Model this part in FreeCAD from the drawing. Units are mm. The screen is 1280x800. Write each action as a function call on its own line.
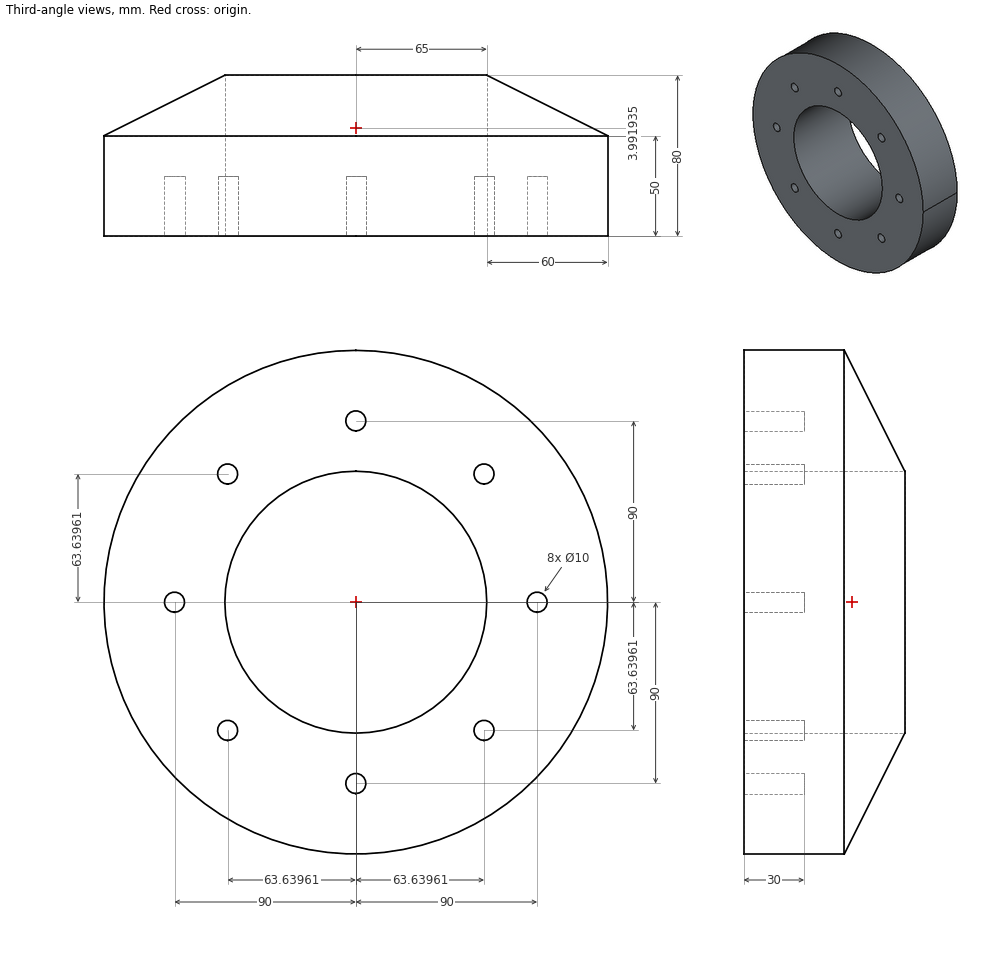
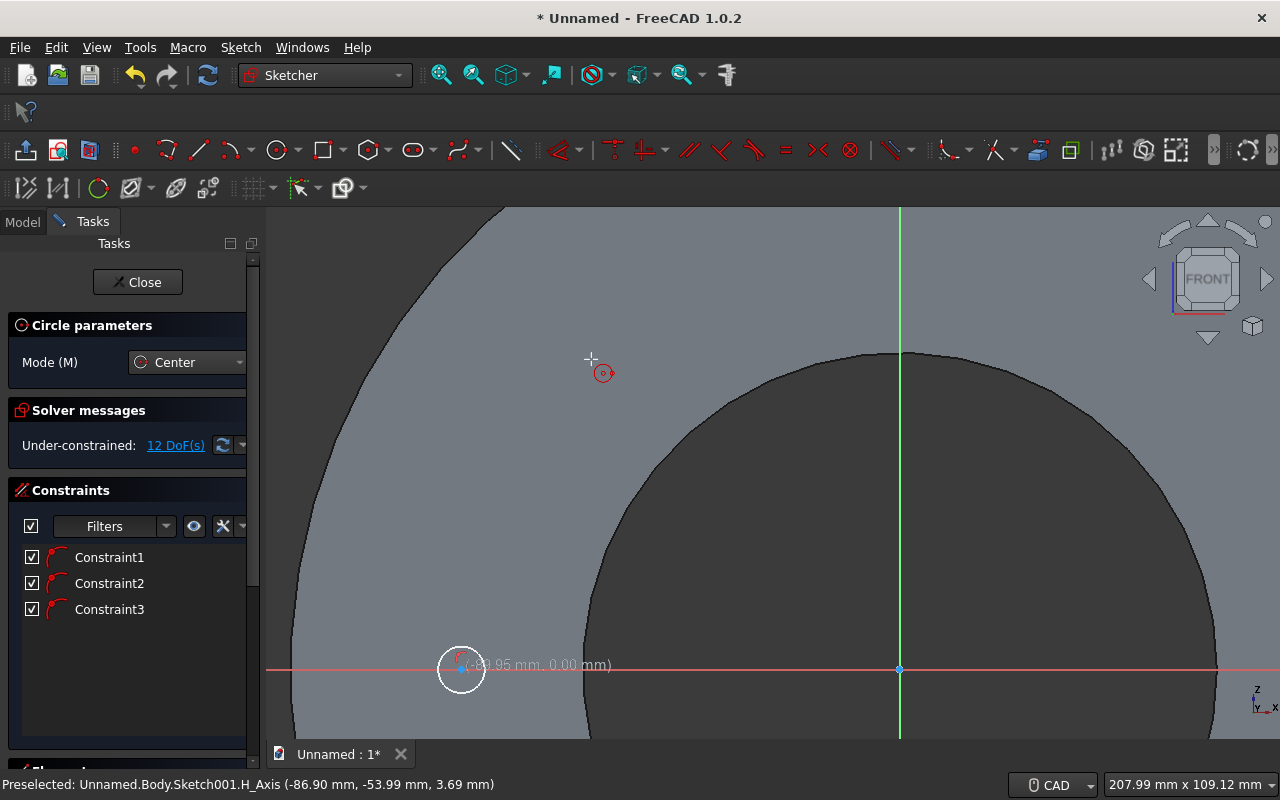
click(590, 360)
click(607, 342)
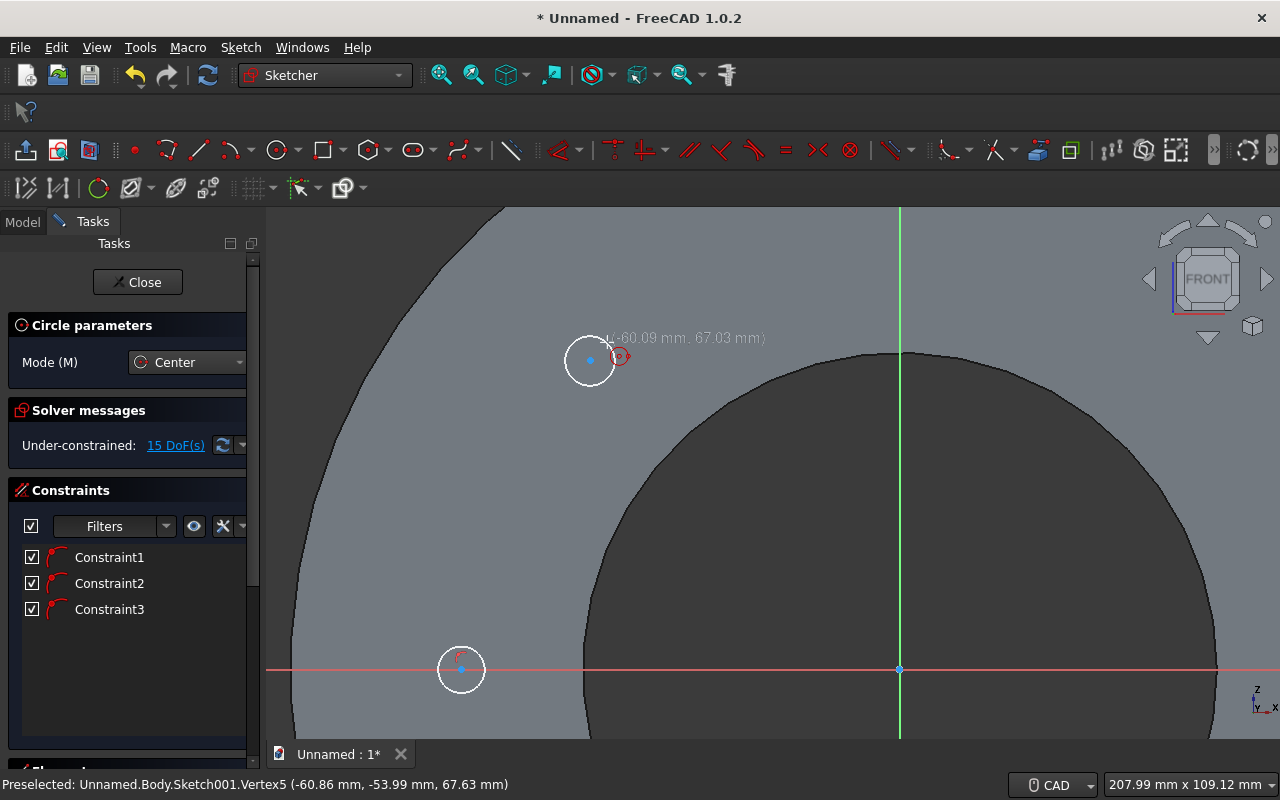
scroll(591, 358, down, 5)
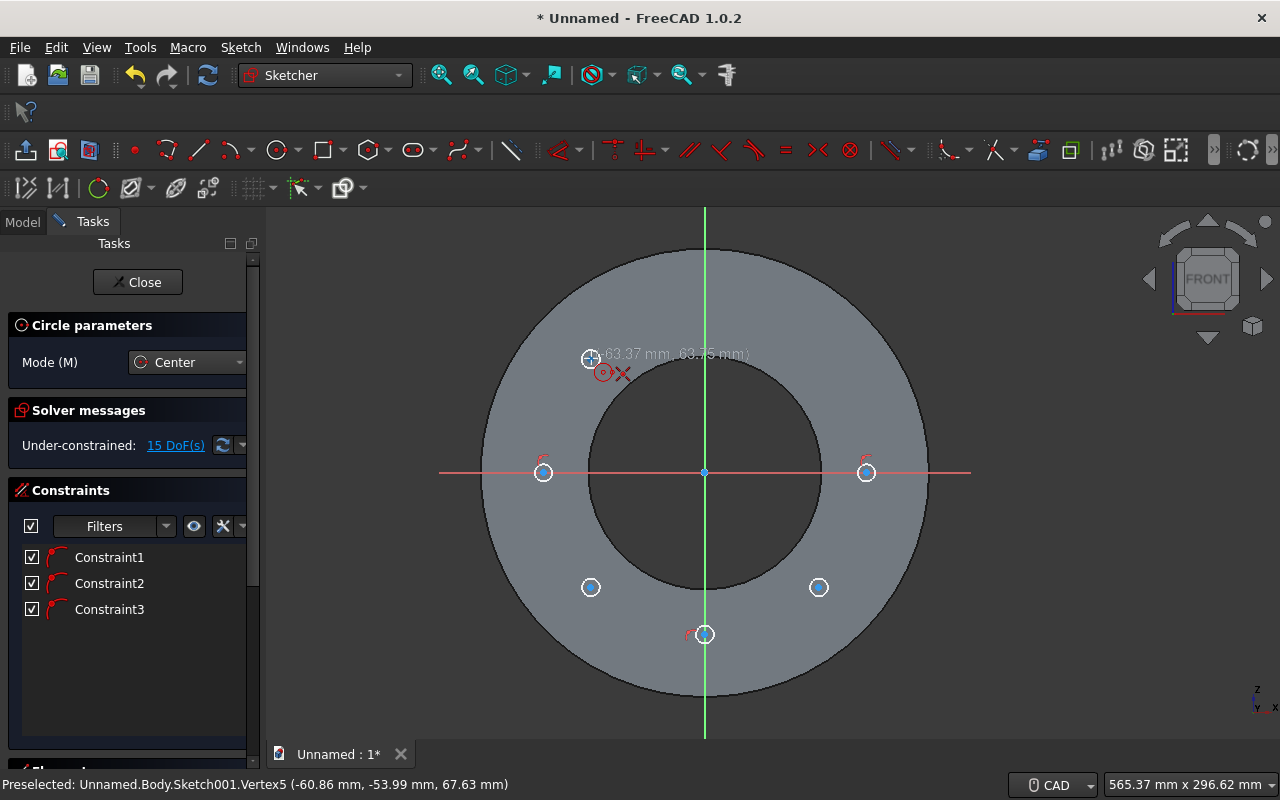
scroll(705, 311, up, 5)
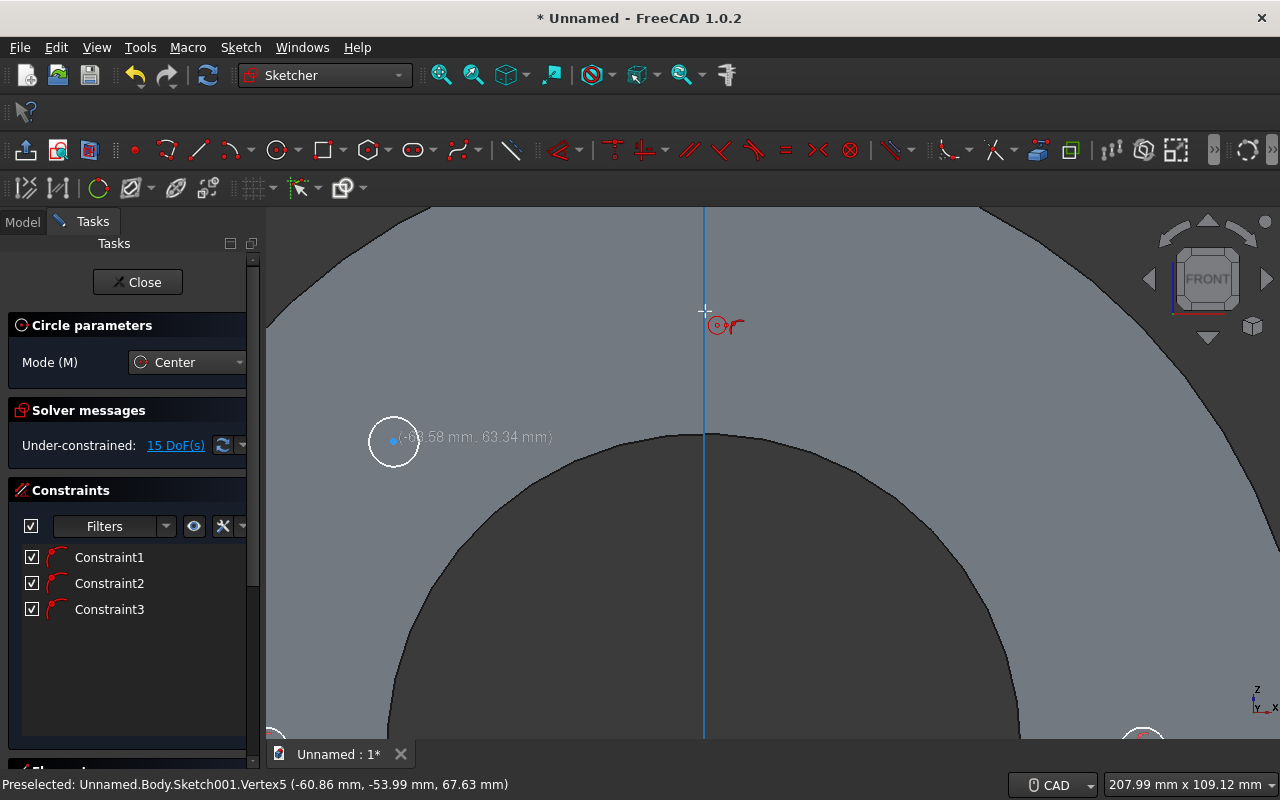
click(704, 312)
click(721, 295)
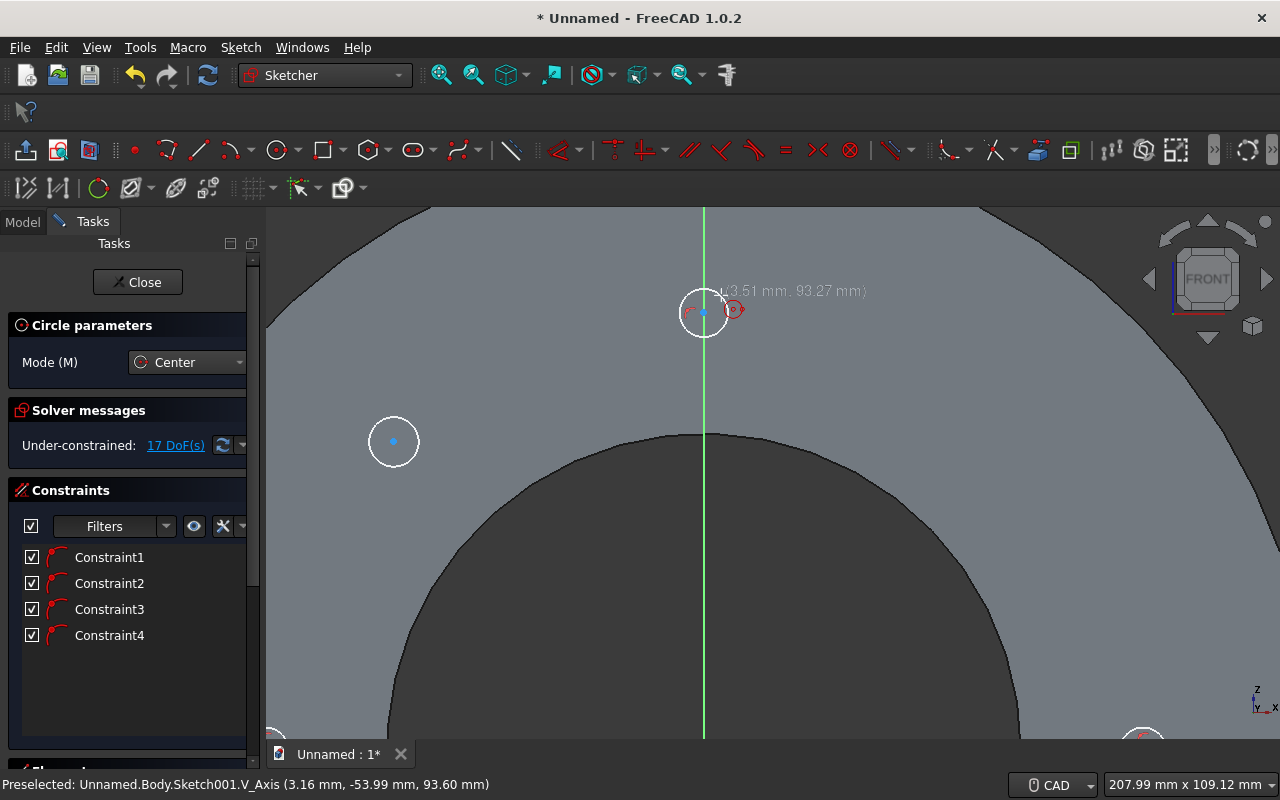
click(1014, 440)
click(1031, 423)
key(Escape)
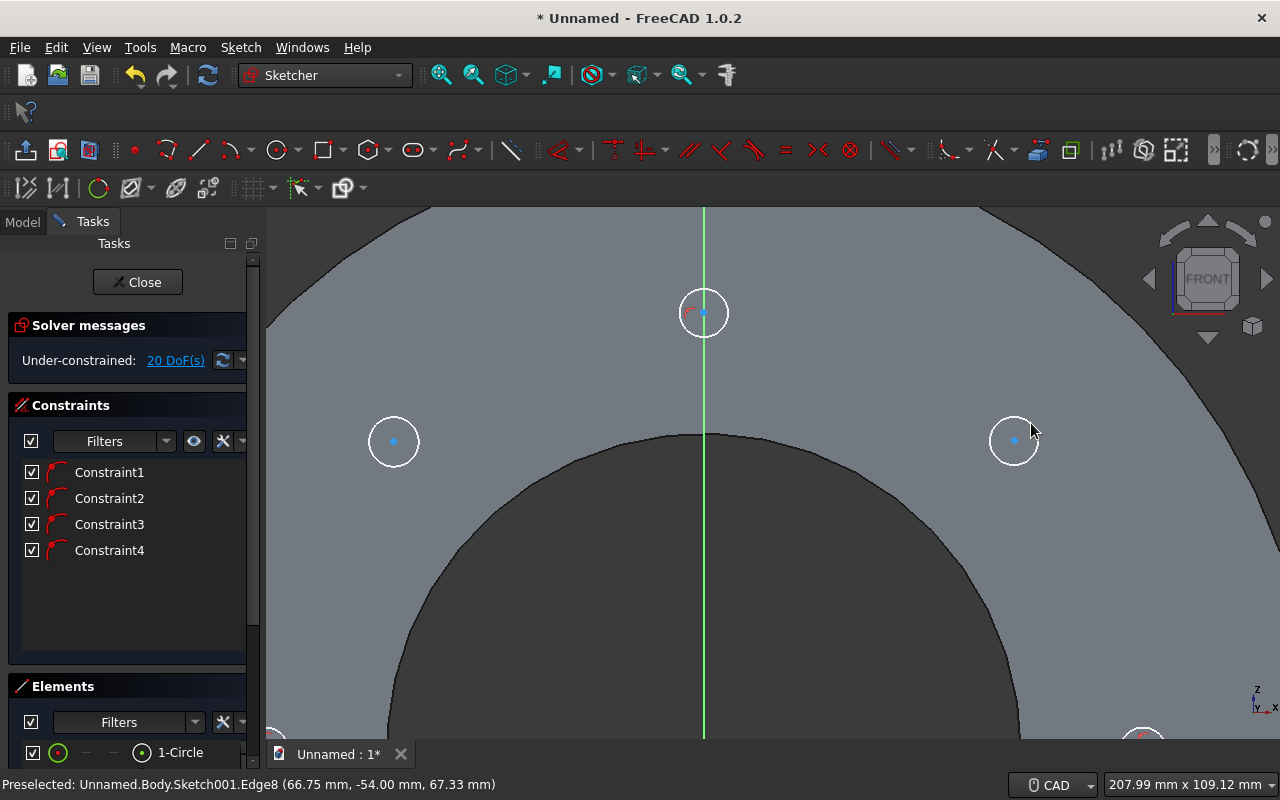
scroll(705, 311, down, 5)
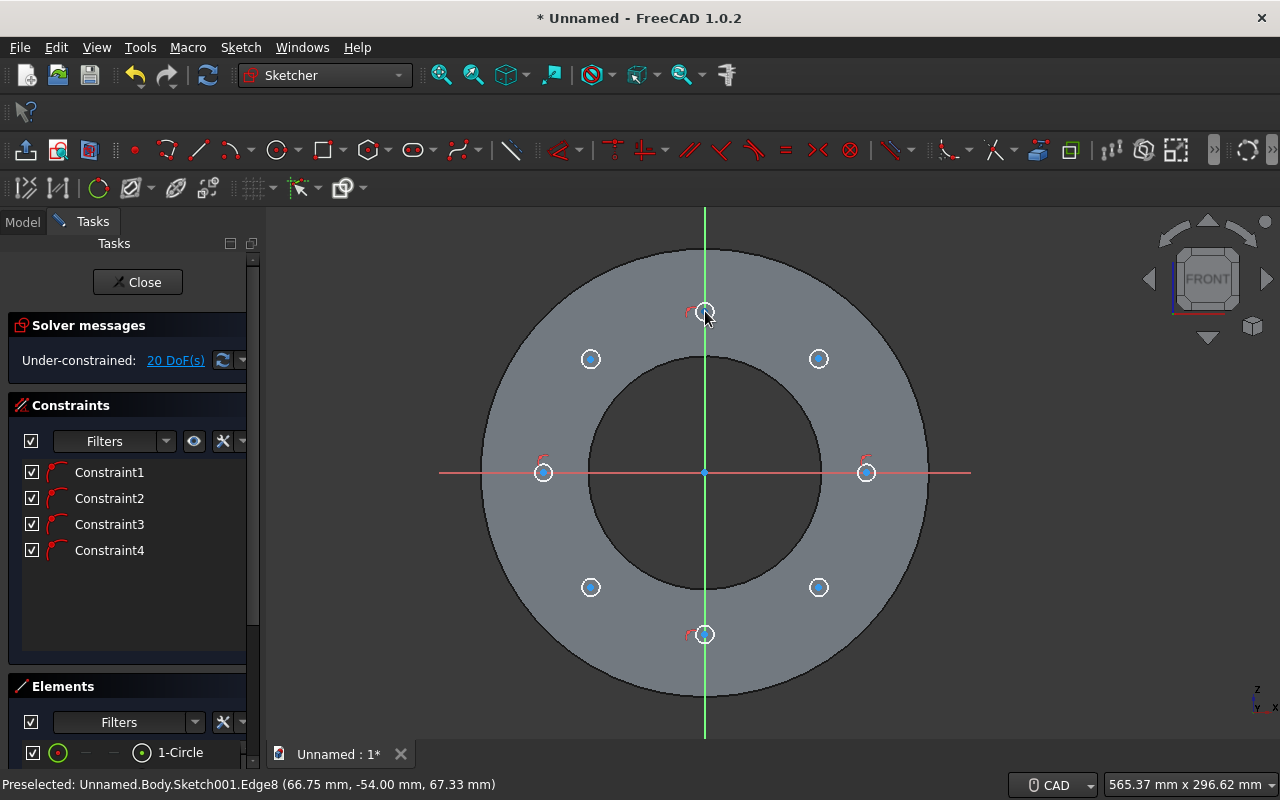
scroll(872, 467, up, 5)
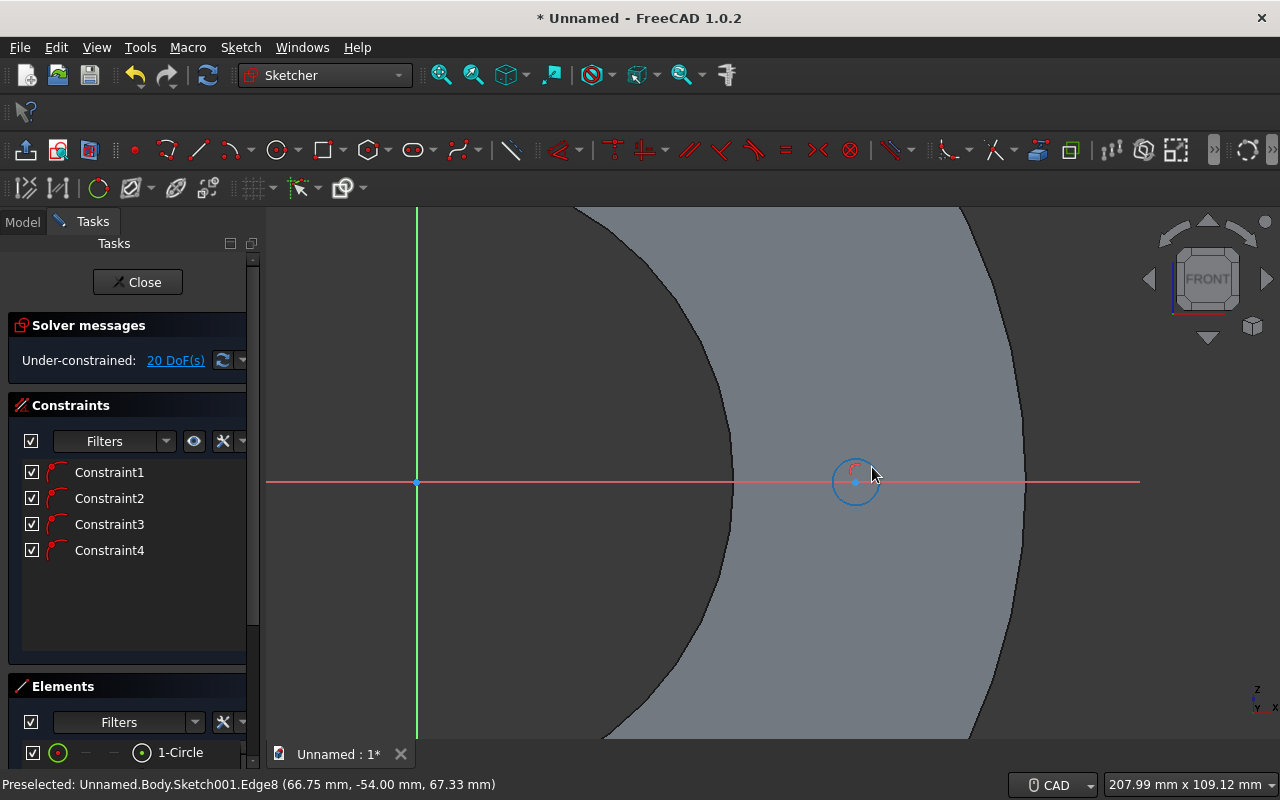
click(872, 466)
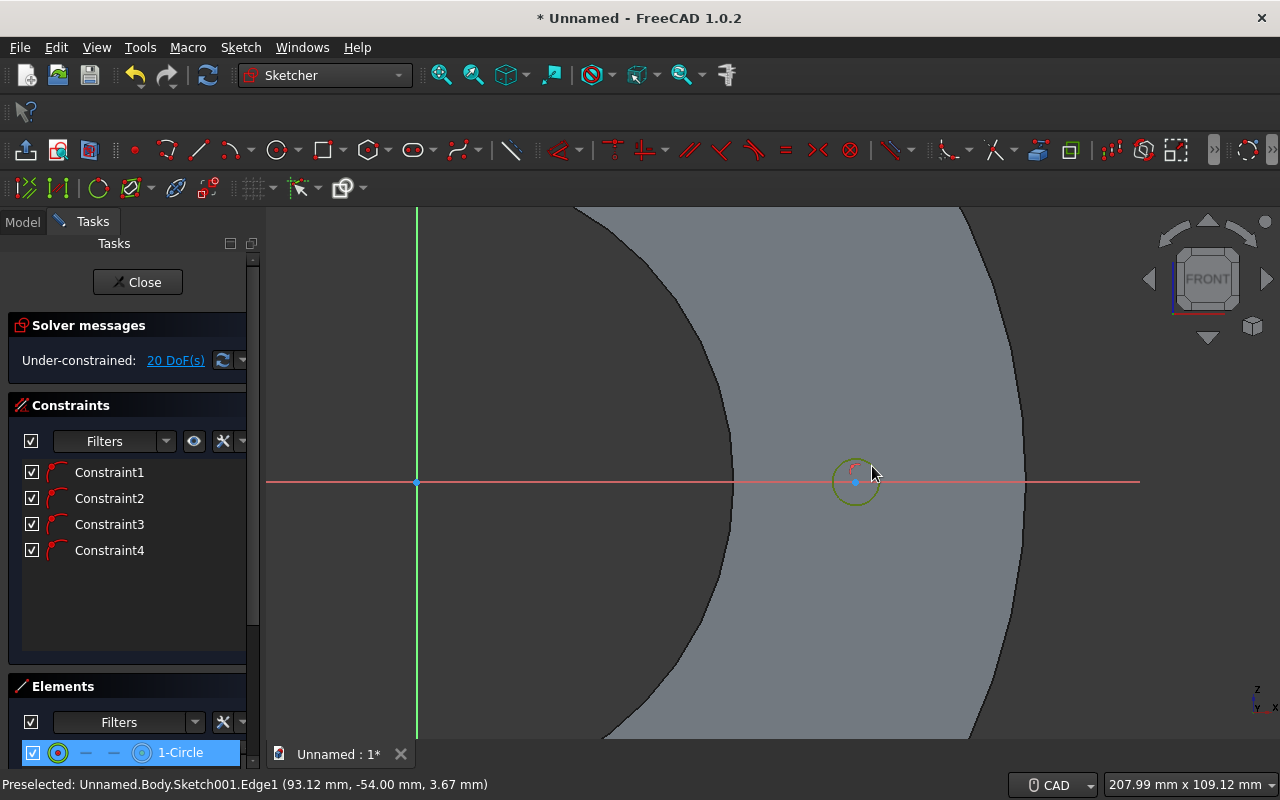
scroll(872, 468, down, 5)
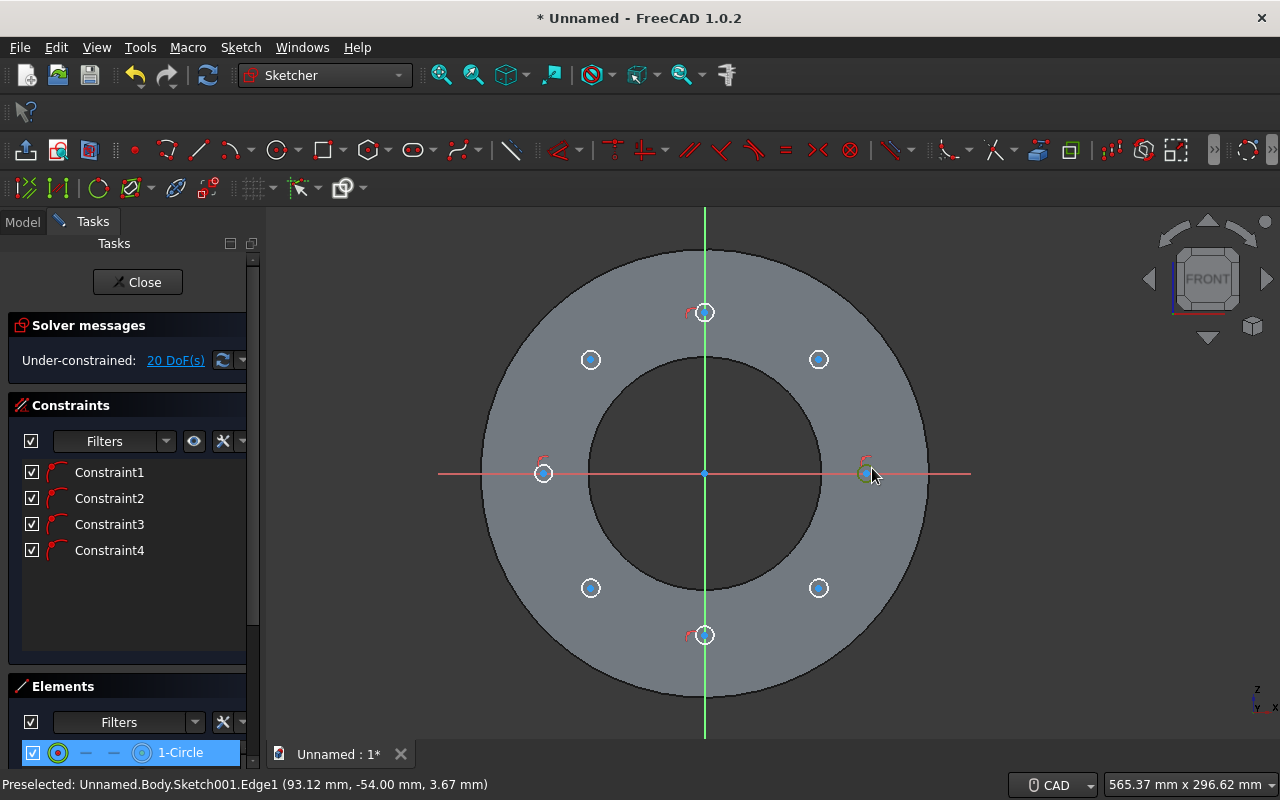
scroll(825, 582, up, 3)